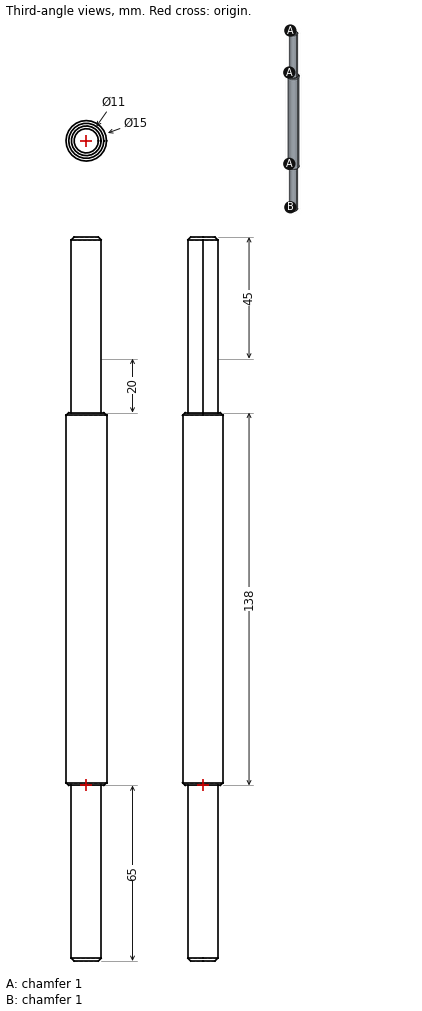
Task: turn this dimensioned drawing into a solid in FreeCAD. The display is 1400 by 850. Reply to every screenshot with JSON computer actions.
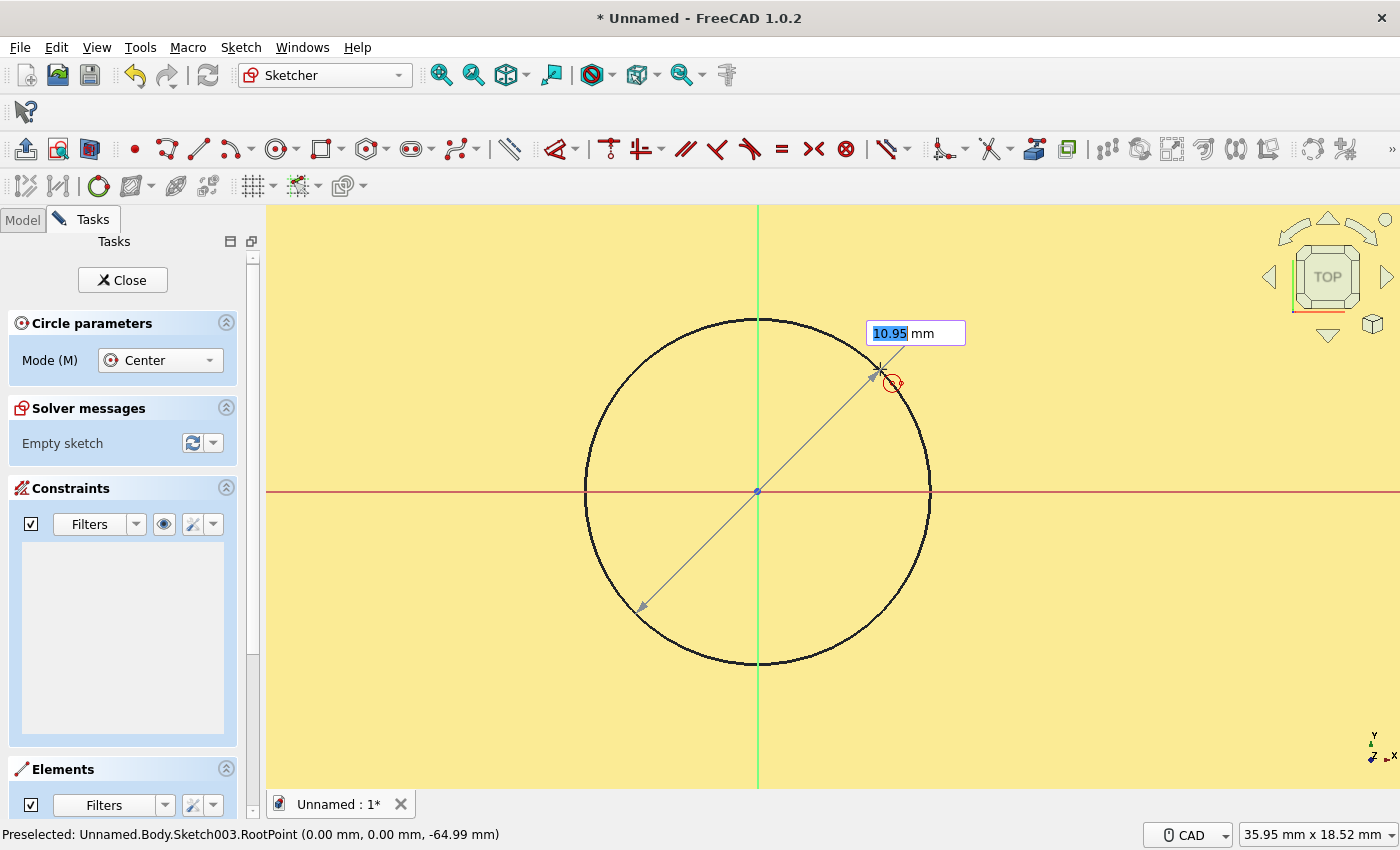
{"action": "type", "text": "11"}
{"action": "key", "text": "Return"}
{"action": "key", "text": "Escape"}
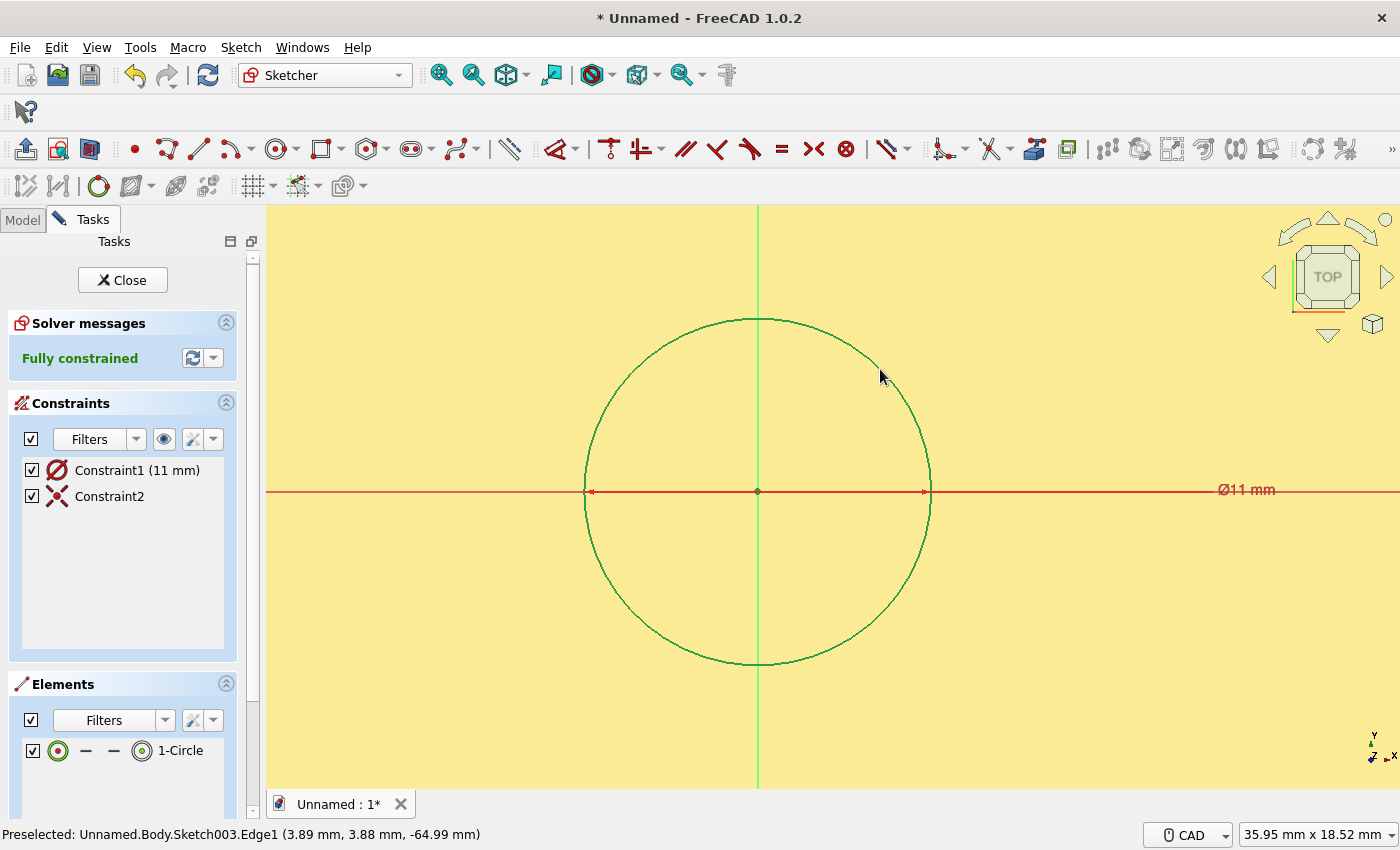
{"action": "left_click", "coordinate": [123, 280]}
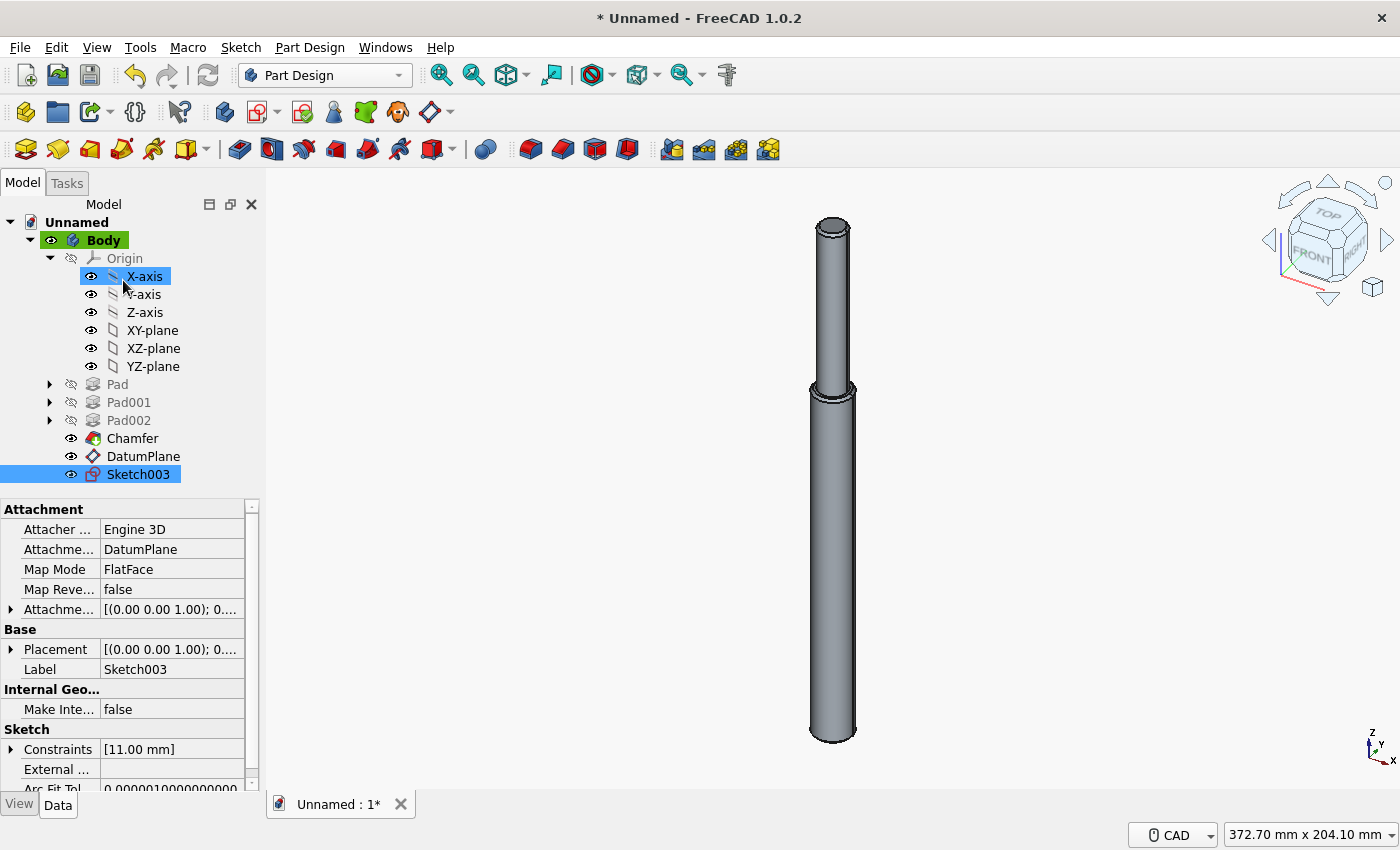
{"action": "left_click", "coordinate": [26, 150]}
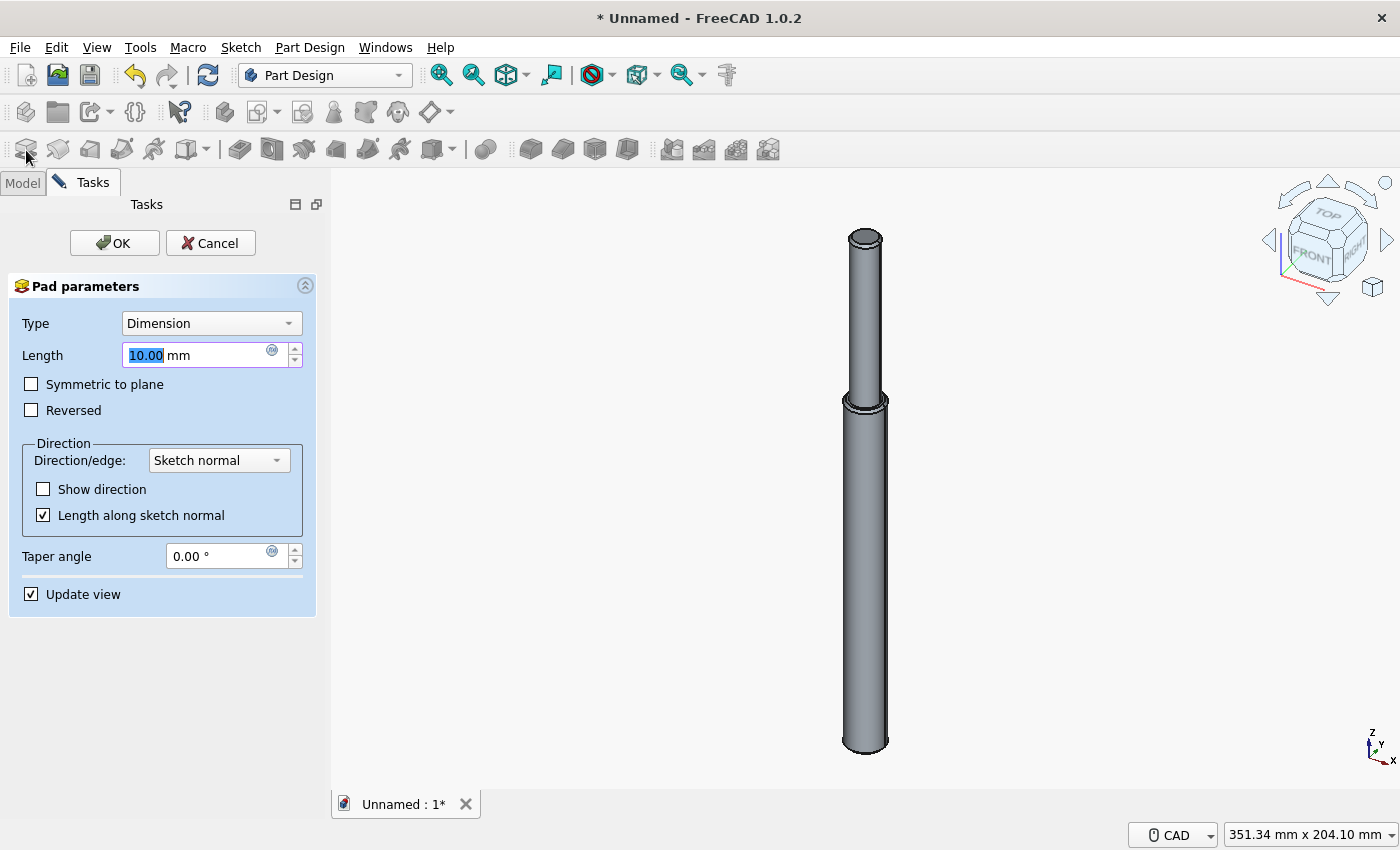
{"action": "type", "text": "65"}
{"action": "key", "text": "Tab"}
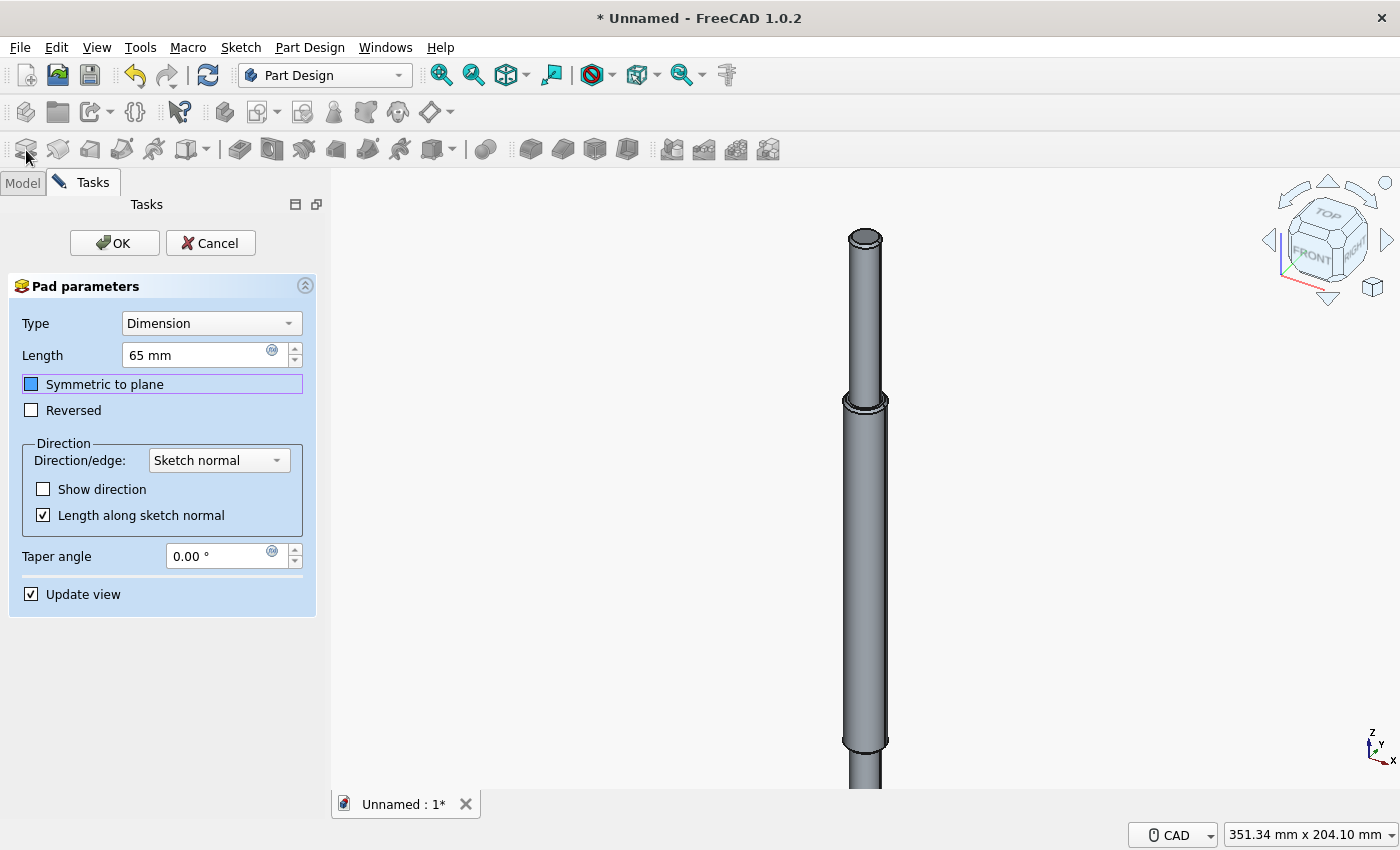
{"action": "left_click", "coordinate": [115, 243]}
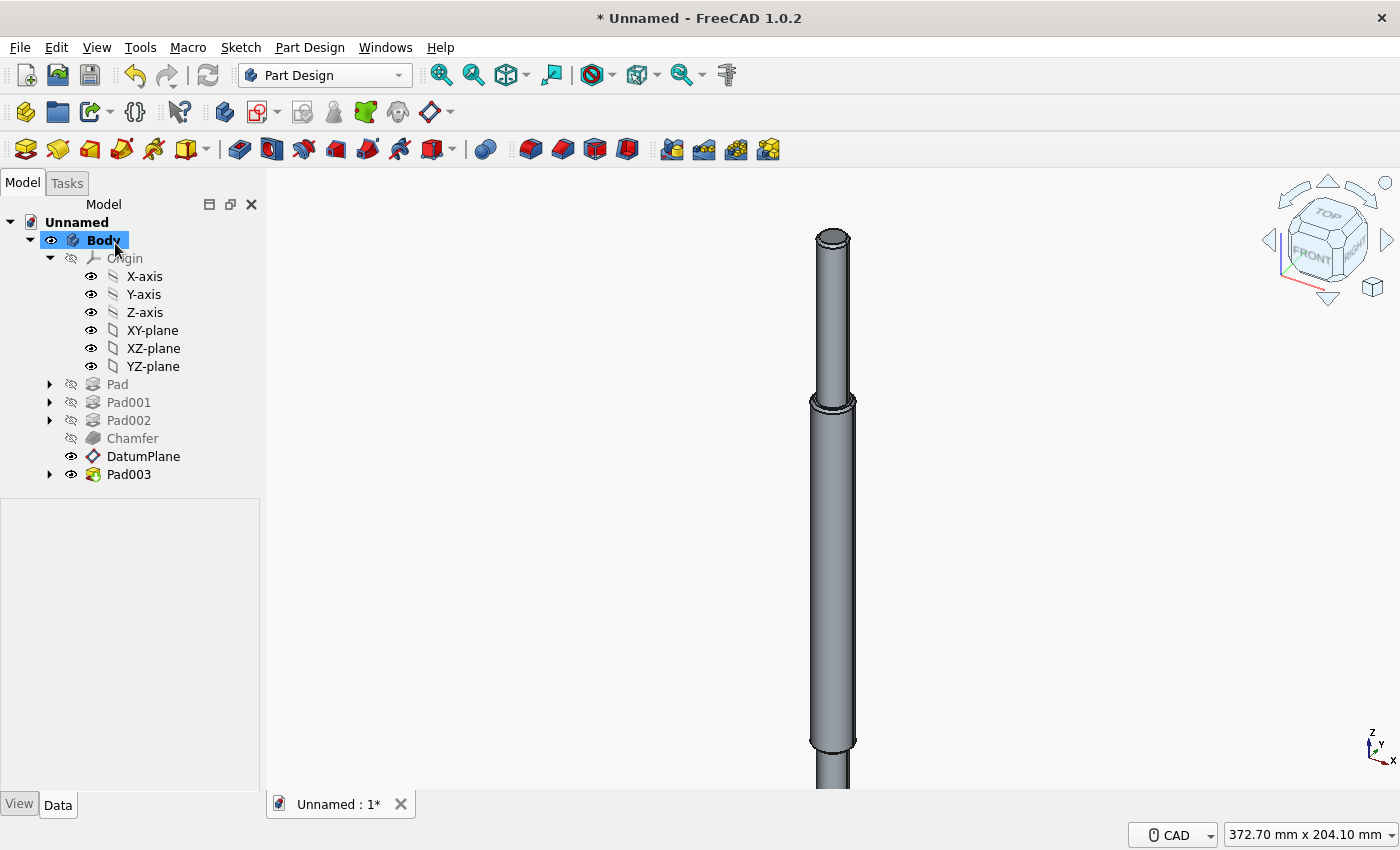
{"action": "left_click", "coordinate": [116, 456]}
{"action": "key", "text": "space"}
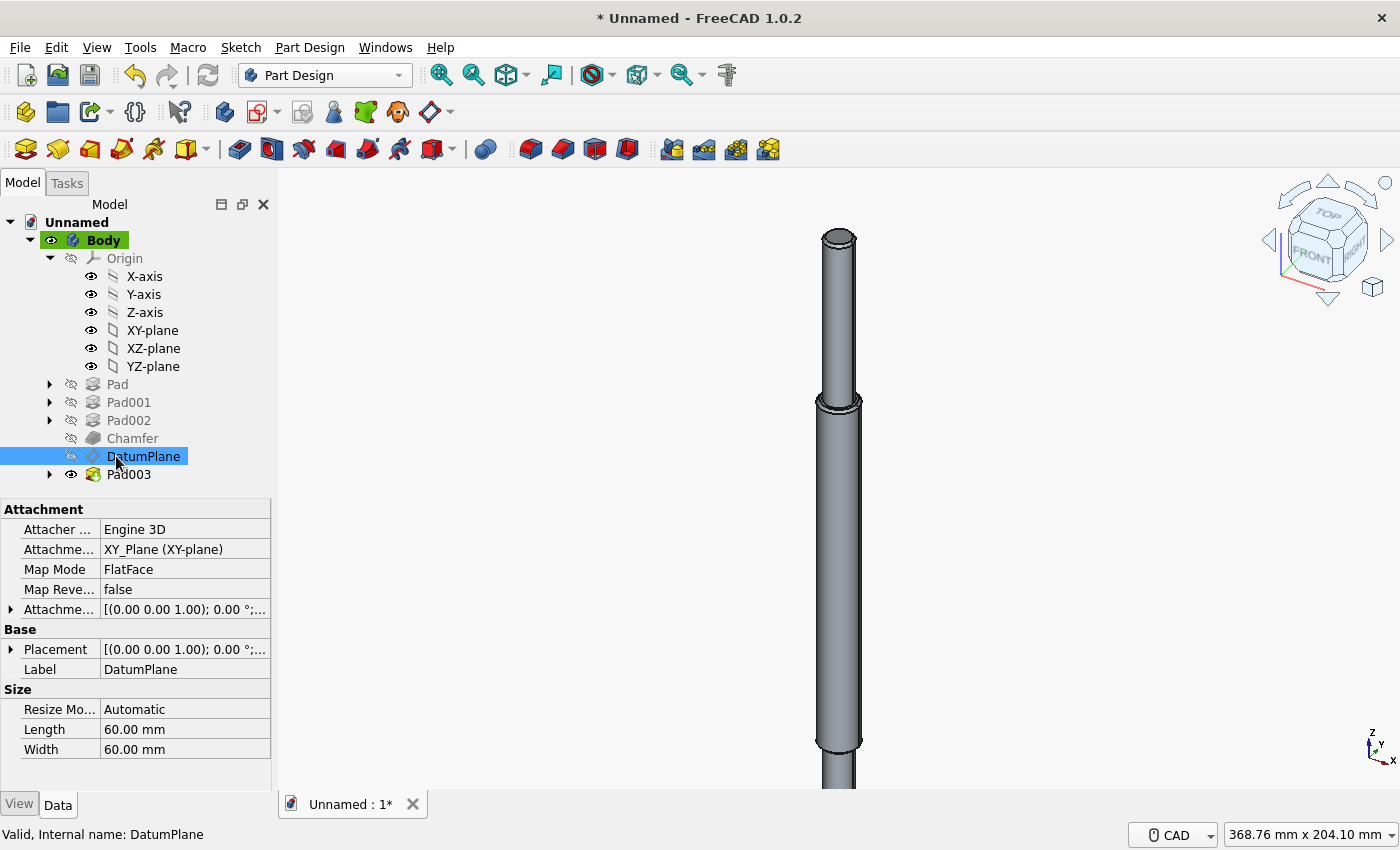
{"action": "key", "text": "v f"}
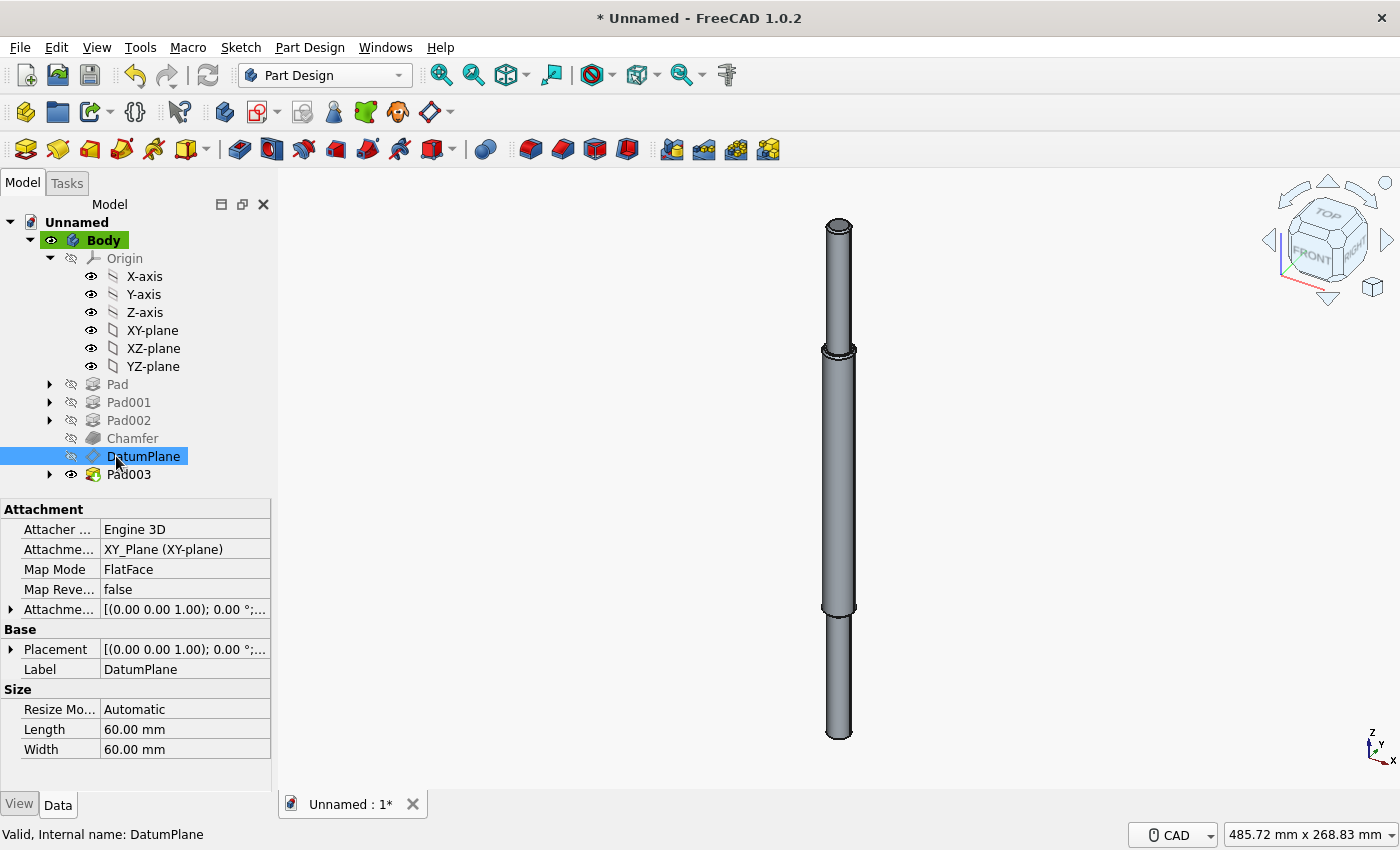
{"action": "left_click", "coordinate": [830, 736]}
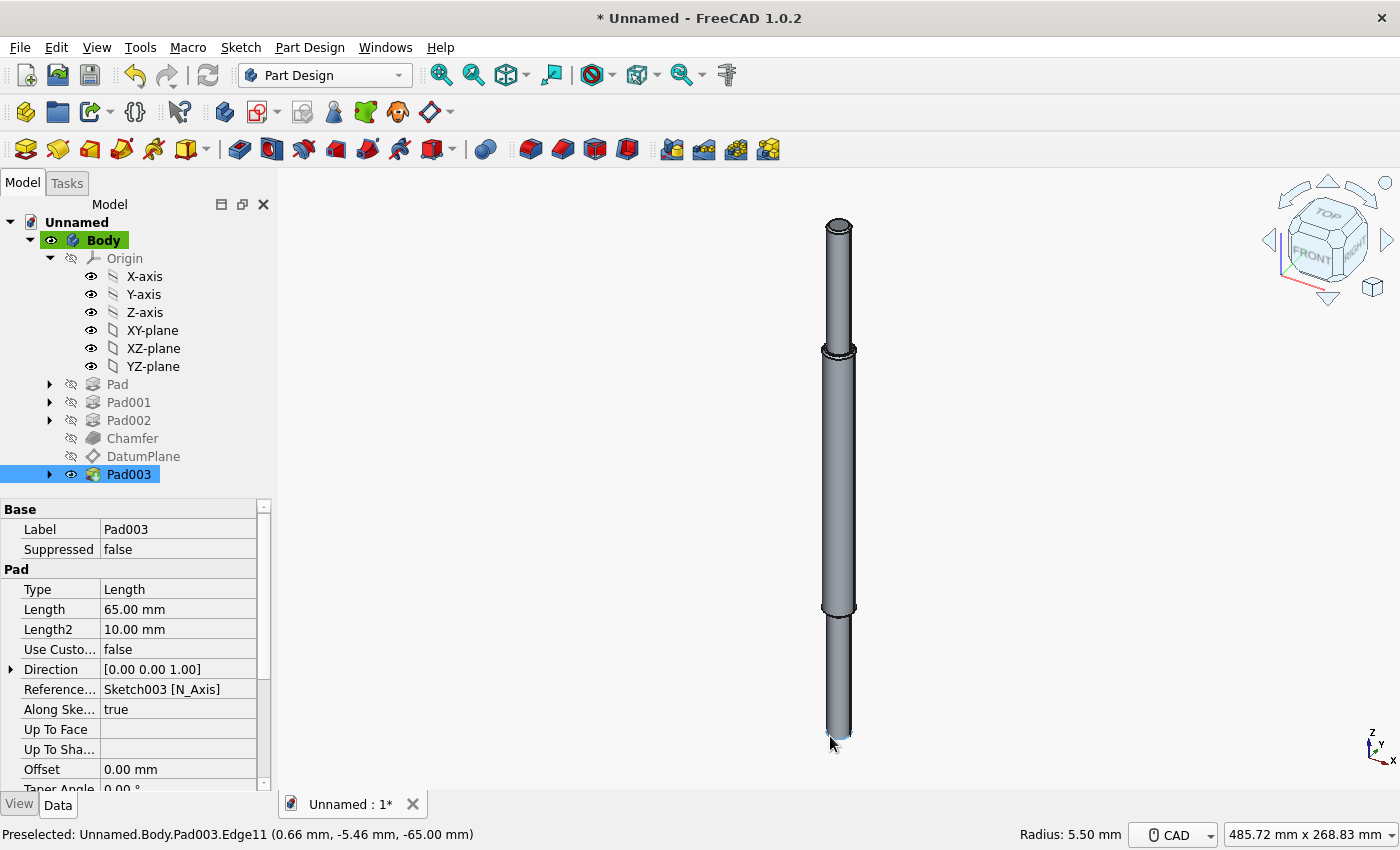
{"action": "left_click", "coordinate": [564, 150]}